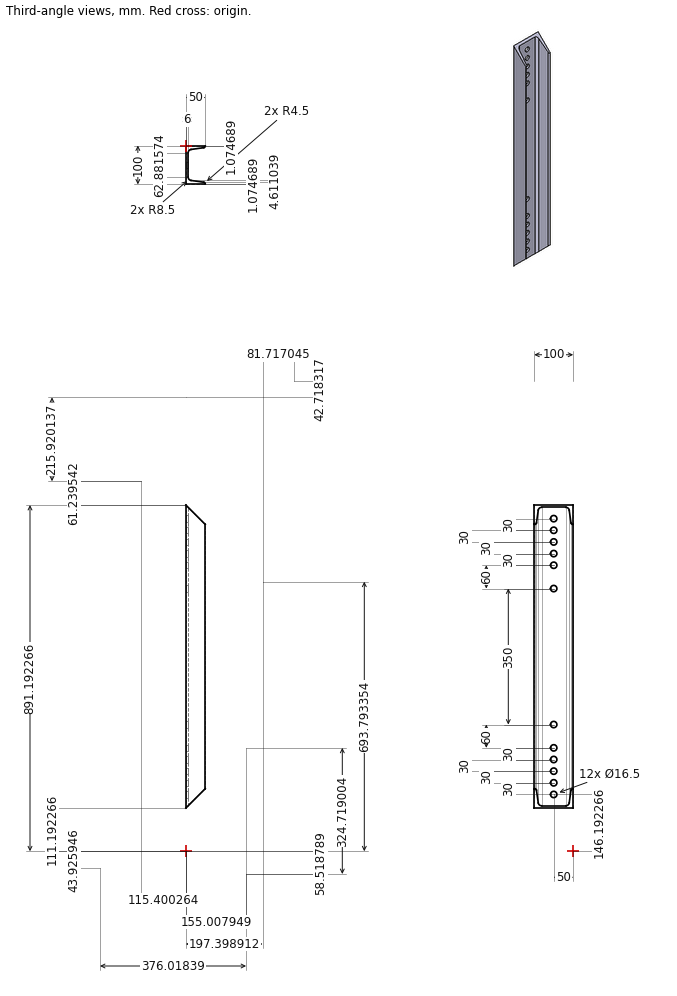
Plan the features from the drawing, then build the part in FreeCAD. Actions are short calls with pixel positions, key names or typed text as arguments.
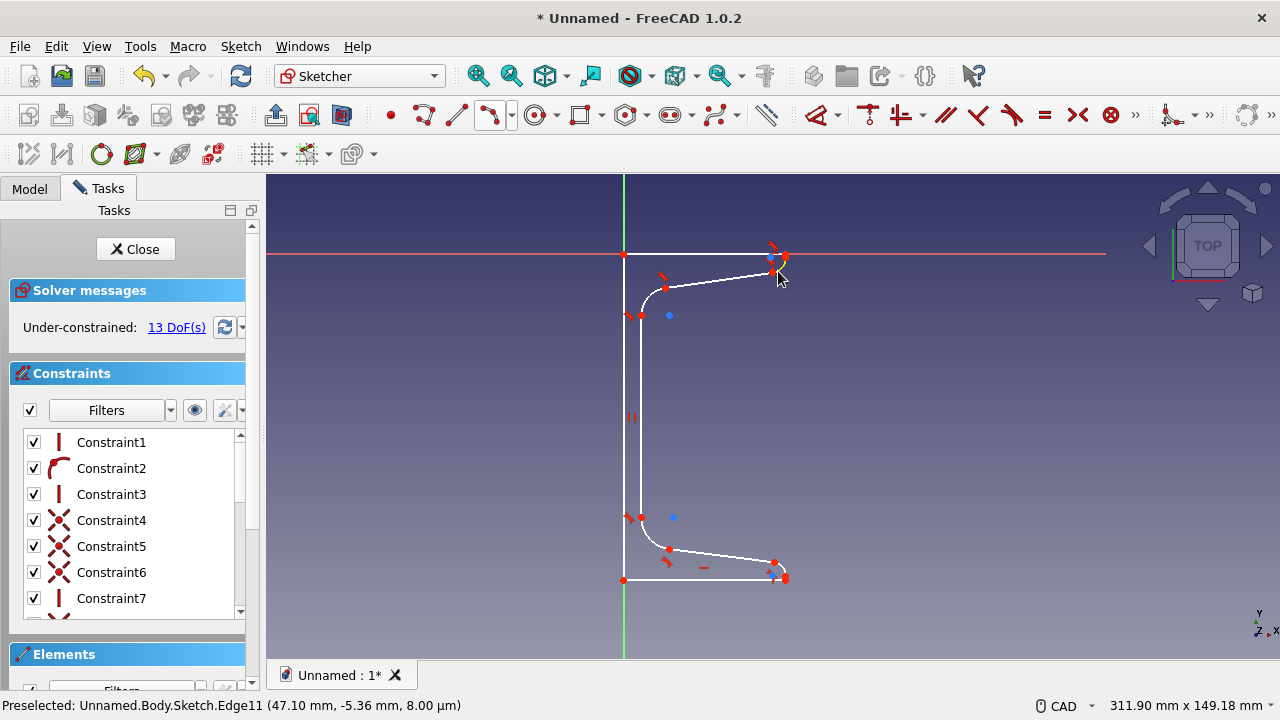
scroll(786, 578, up, 10)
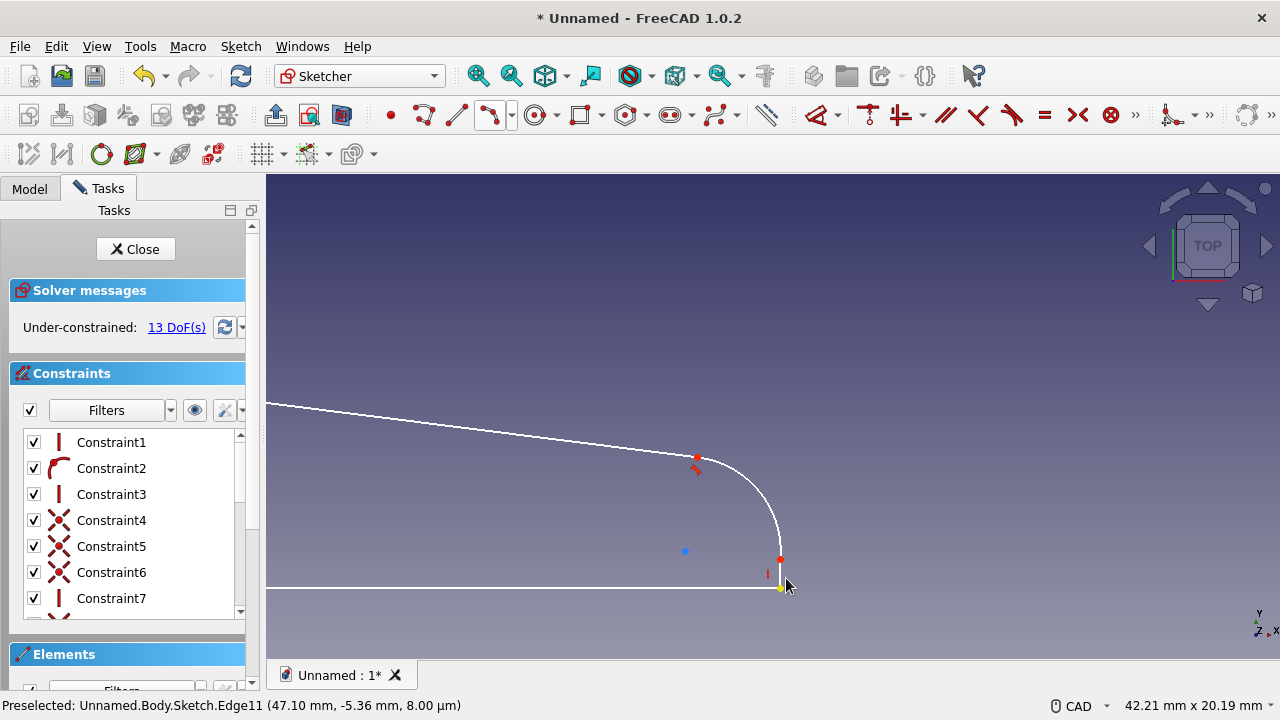
click(780, 574)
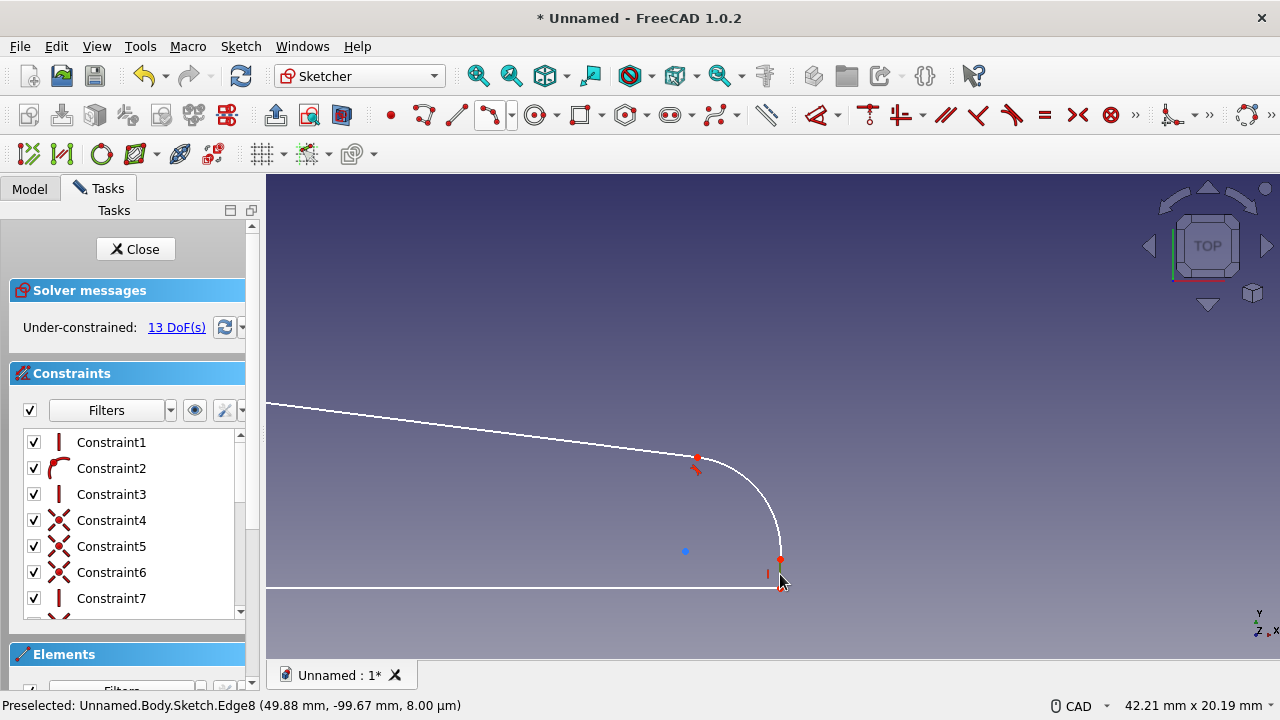
scroll(786, 578, down, 10)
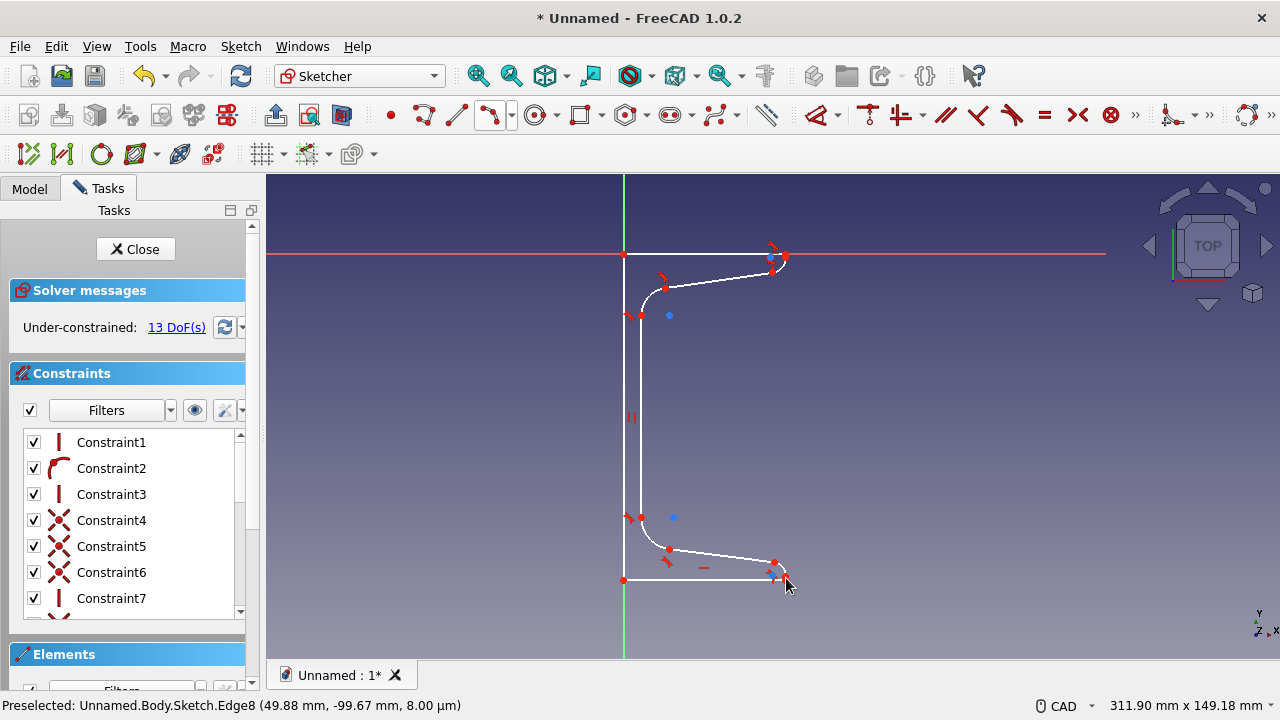
scroll(785, 570, up, 5)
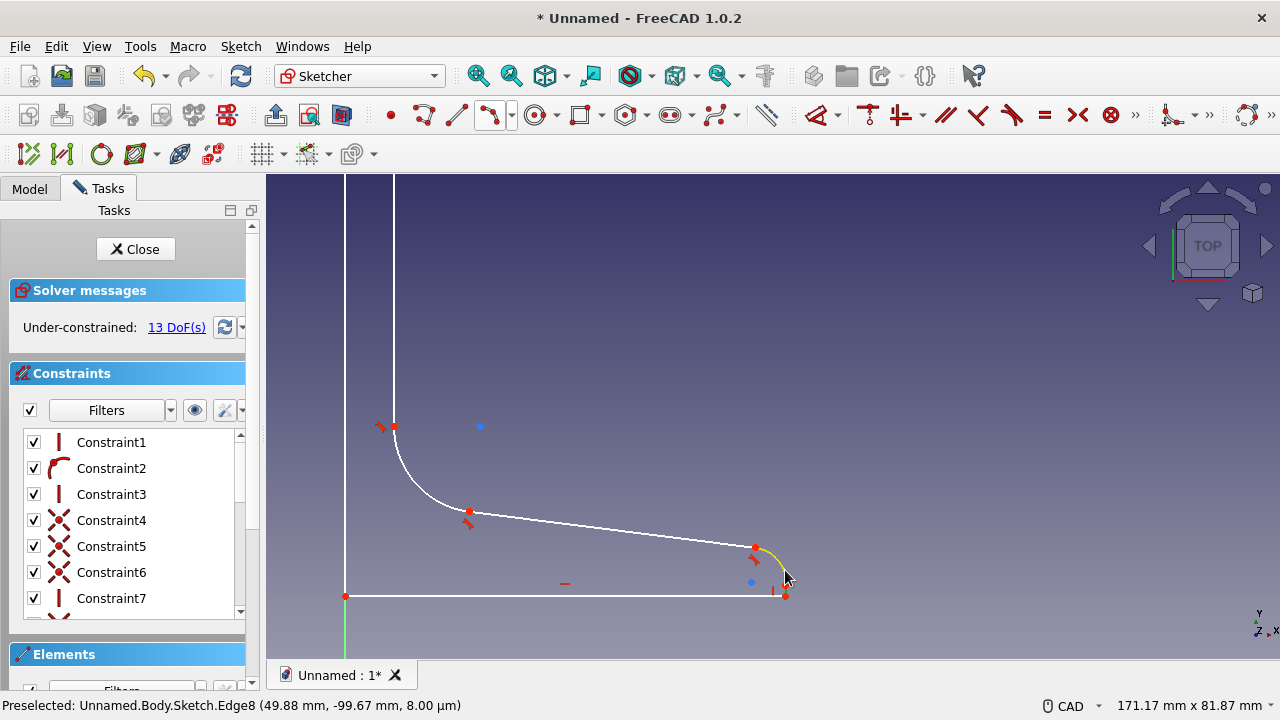
click(784, 570)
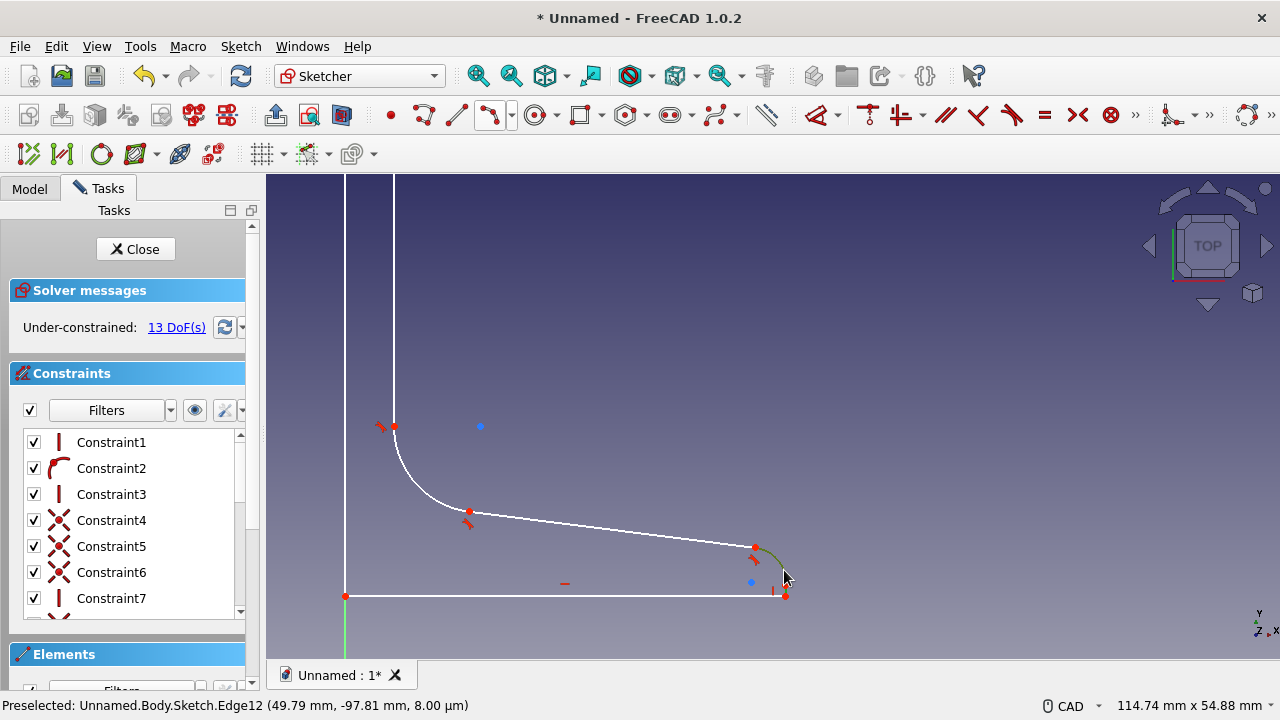
click(1012, 116)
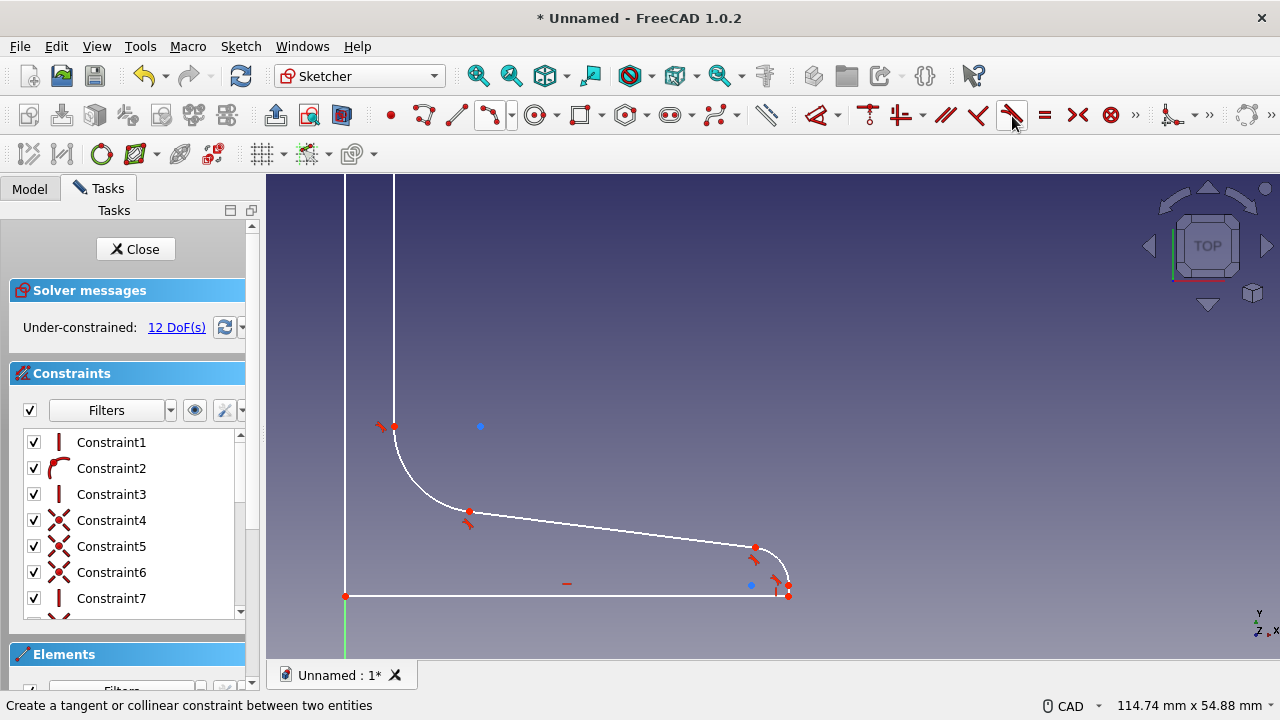
click(402, 462)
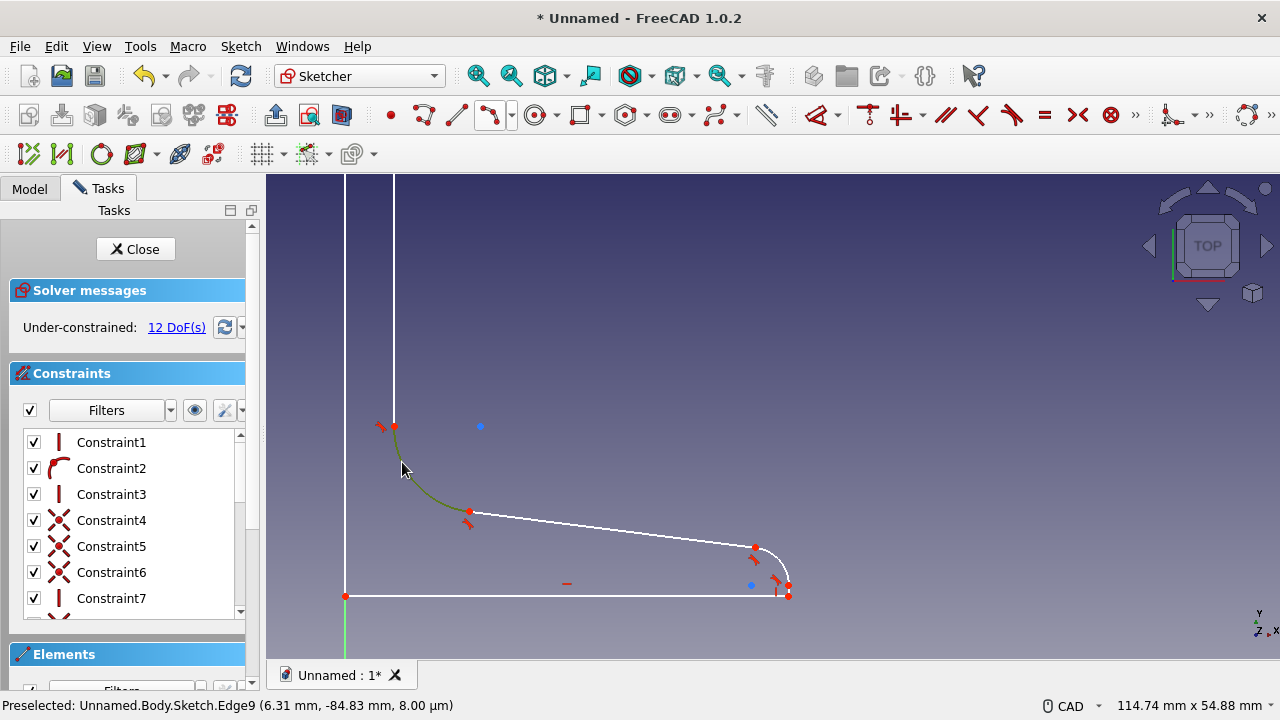
scroll(785, 570, down, 5)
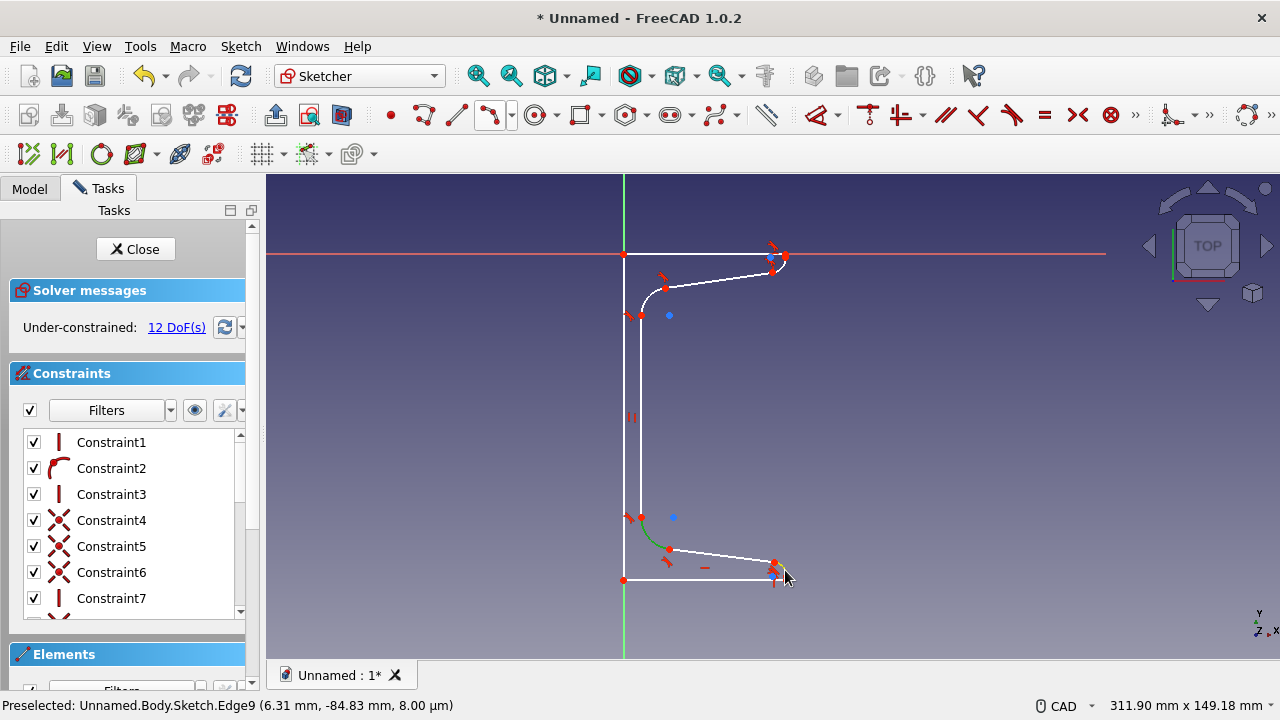
click(654, 292)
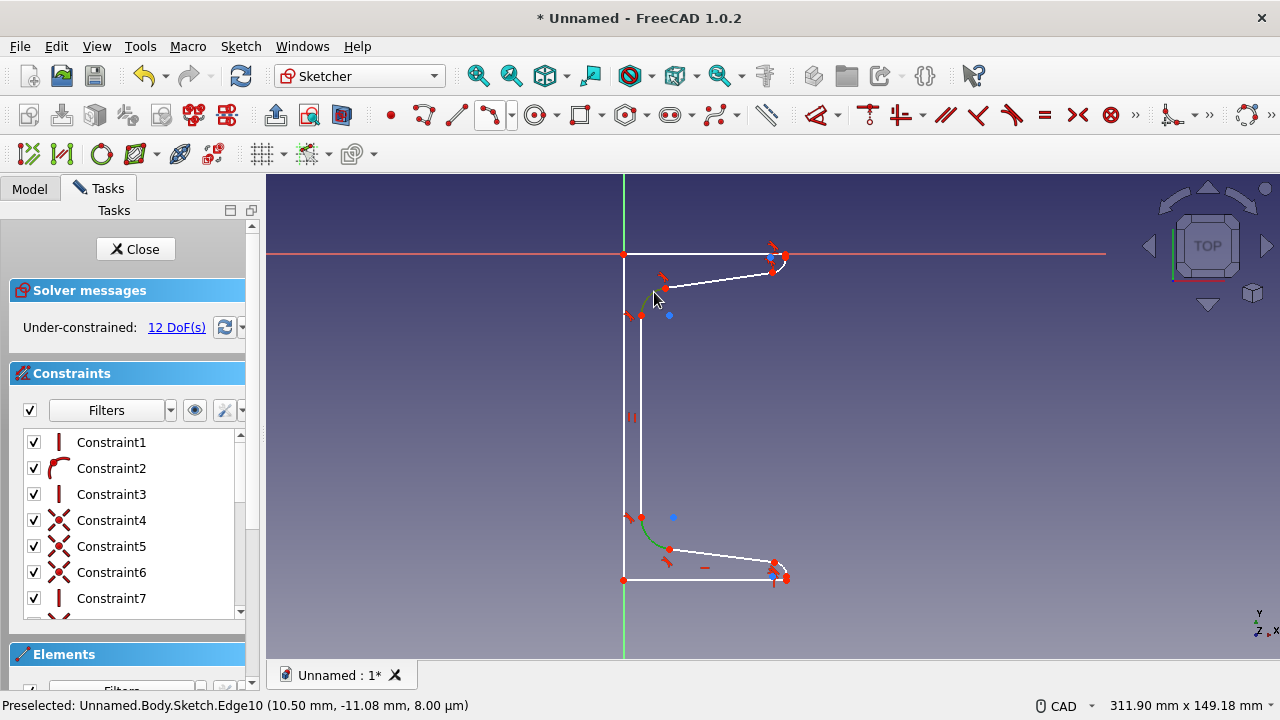
click(1045, 116)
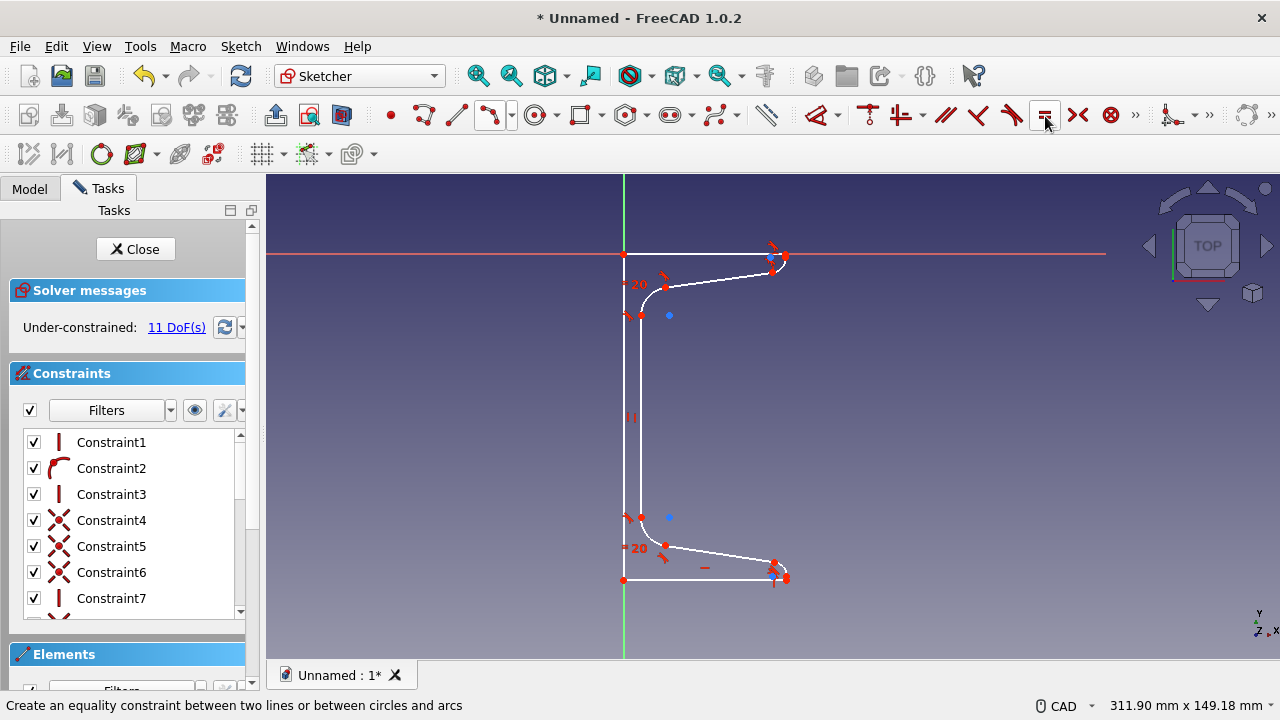
scroll(782, 268, up, 2)